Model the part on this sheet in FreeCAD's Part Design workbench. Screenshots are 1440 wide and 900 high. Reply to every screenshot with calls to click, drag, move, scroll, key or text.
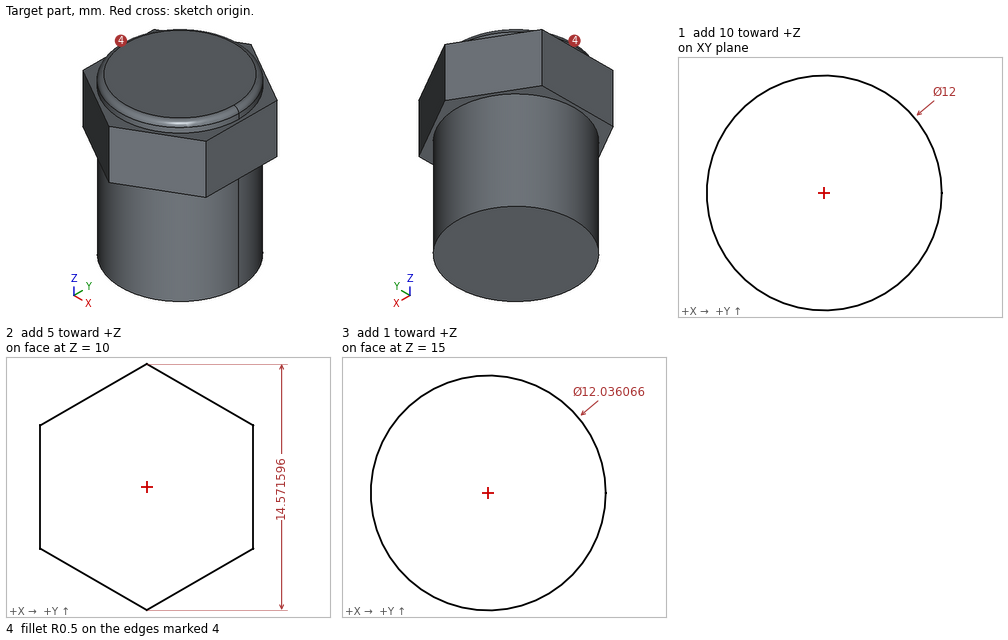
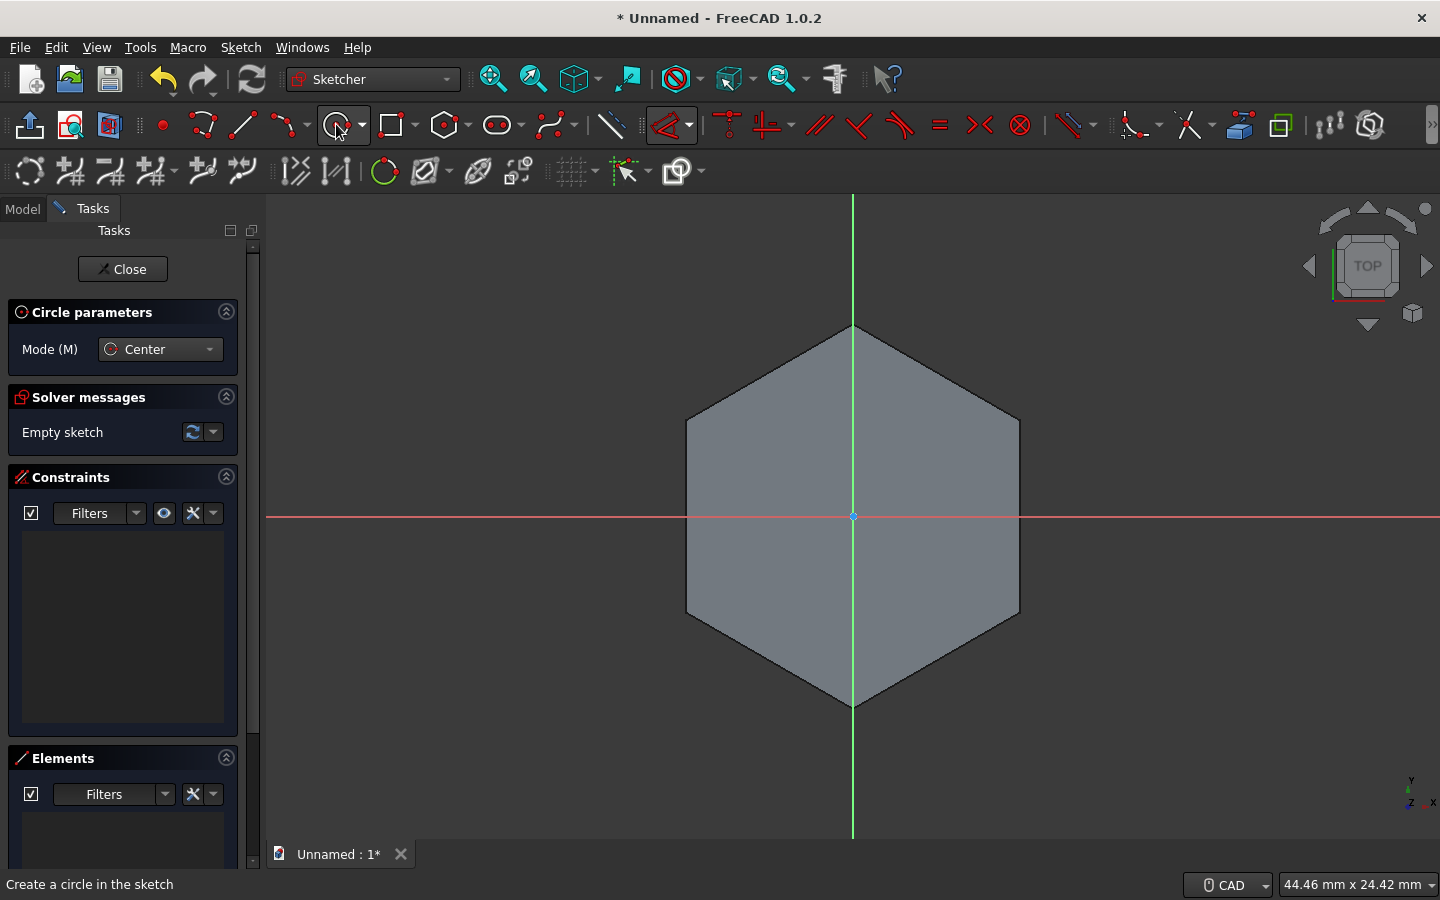
click(853, 516)
click(965, 404)
key(Escape)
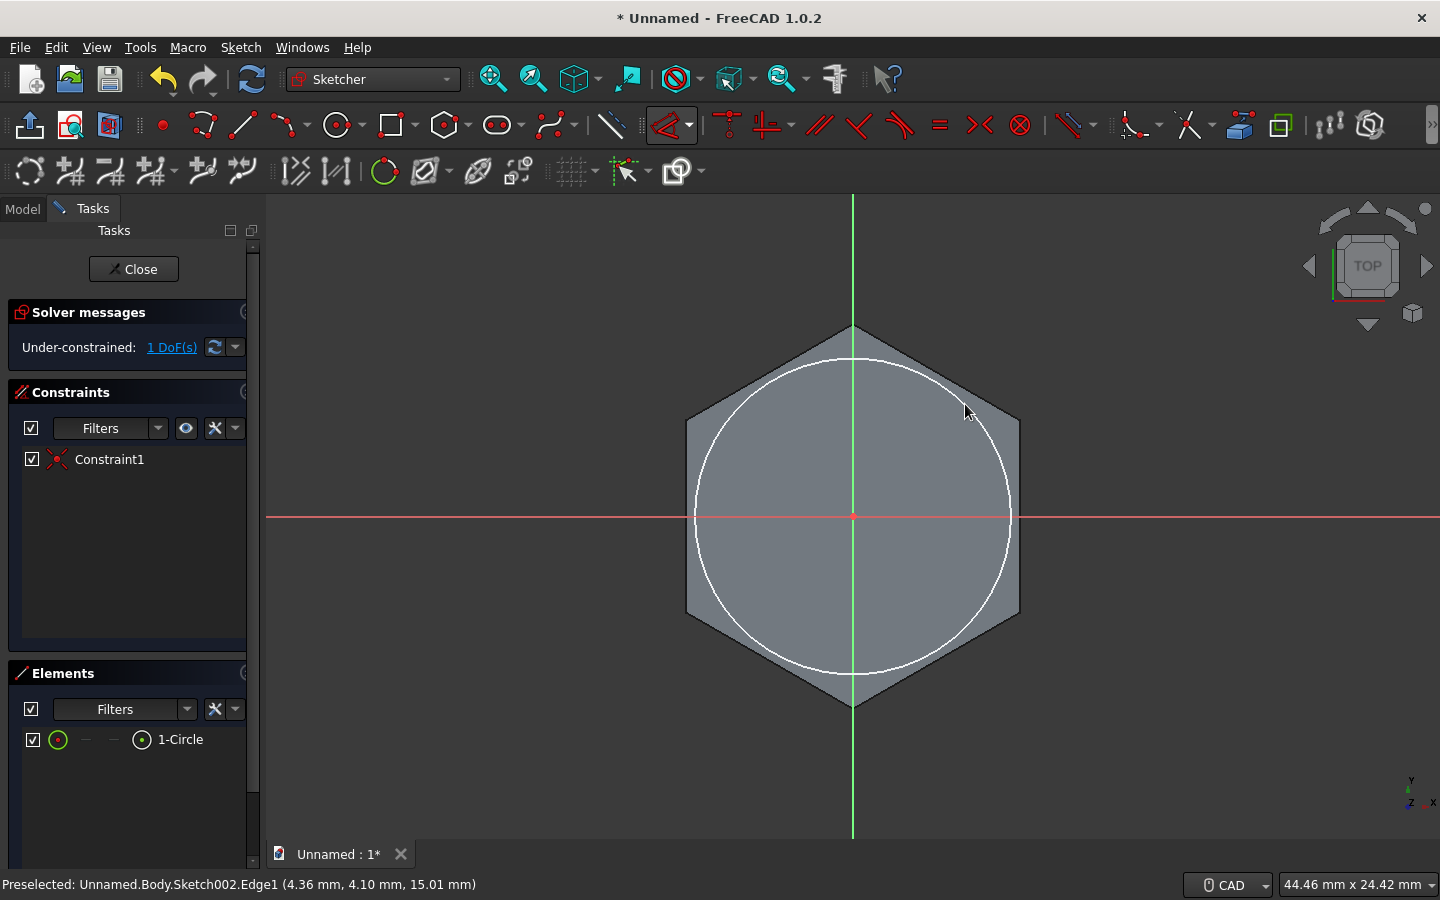
click(964, 404)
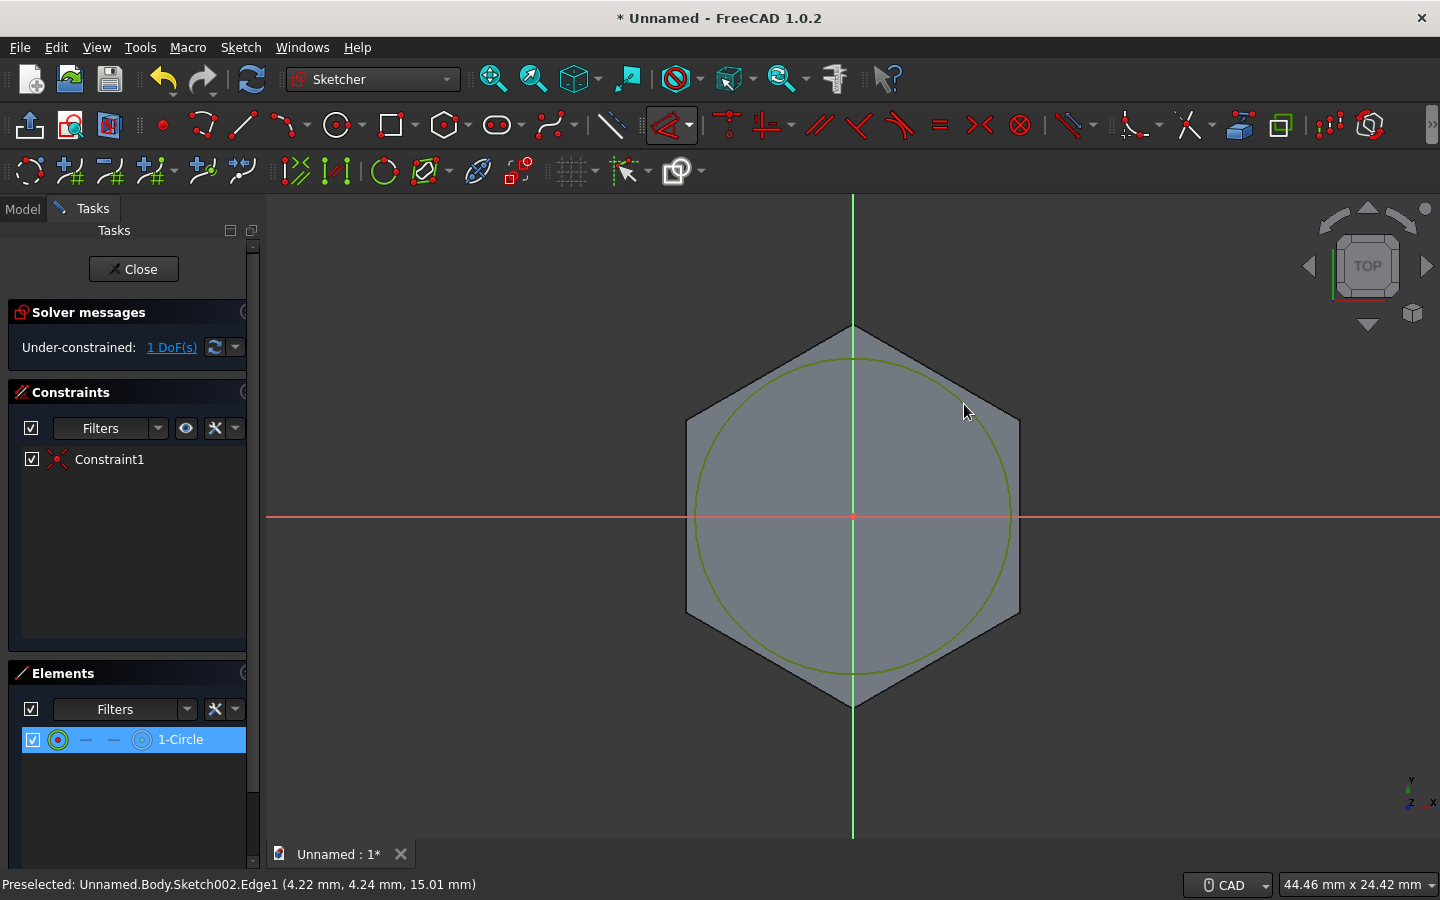
click(692, 126)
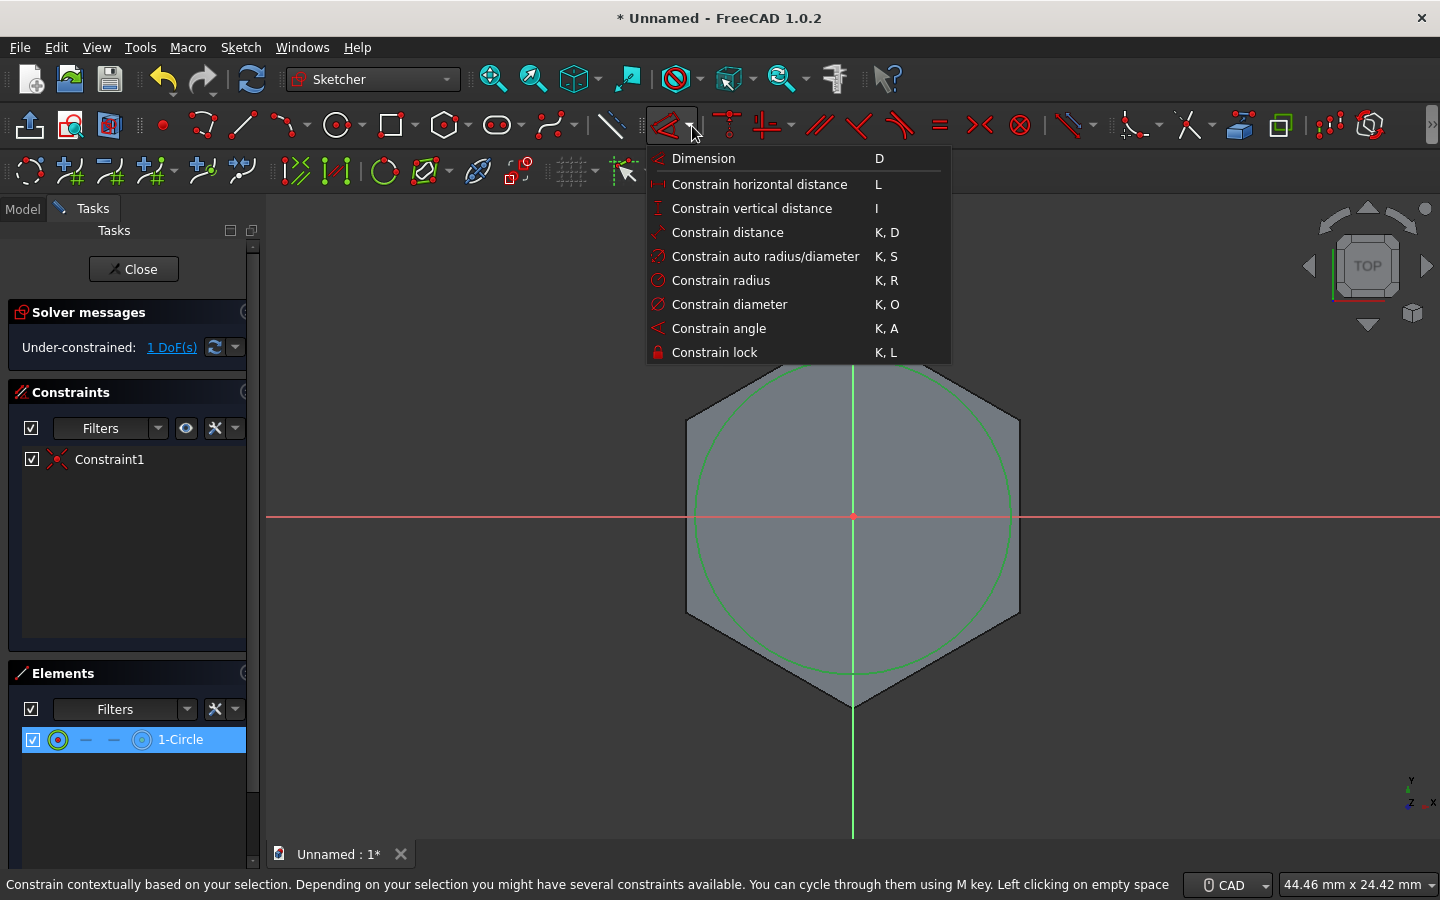
click(799, 304)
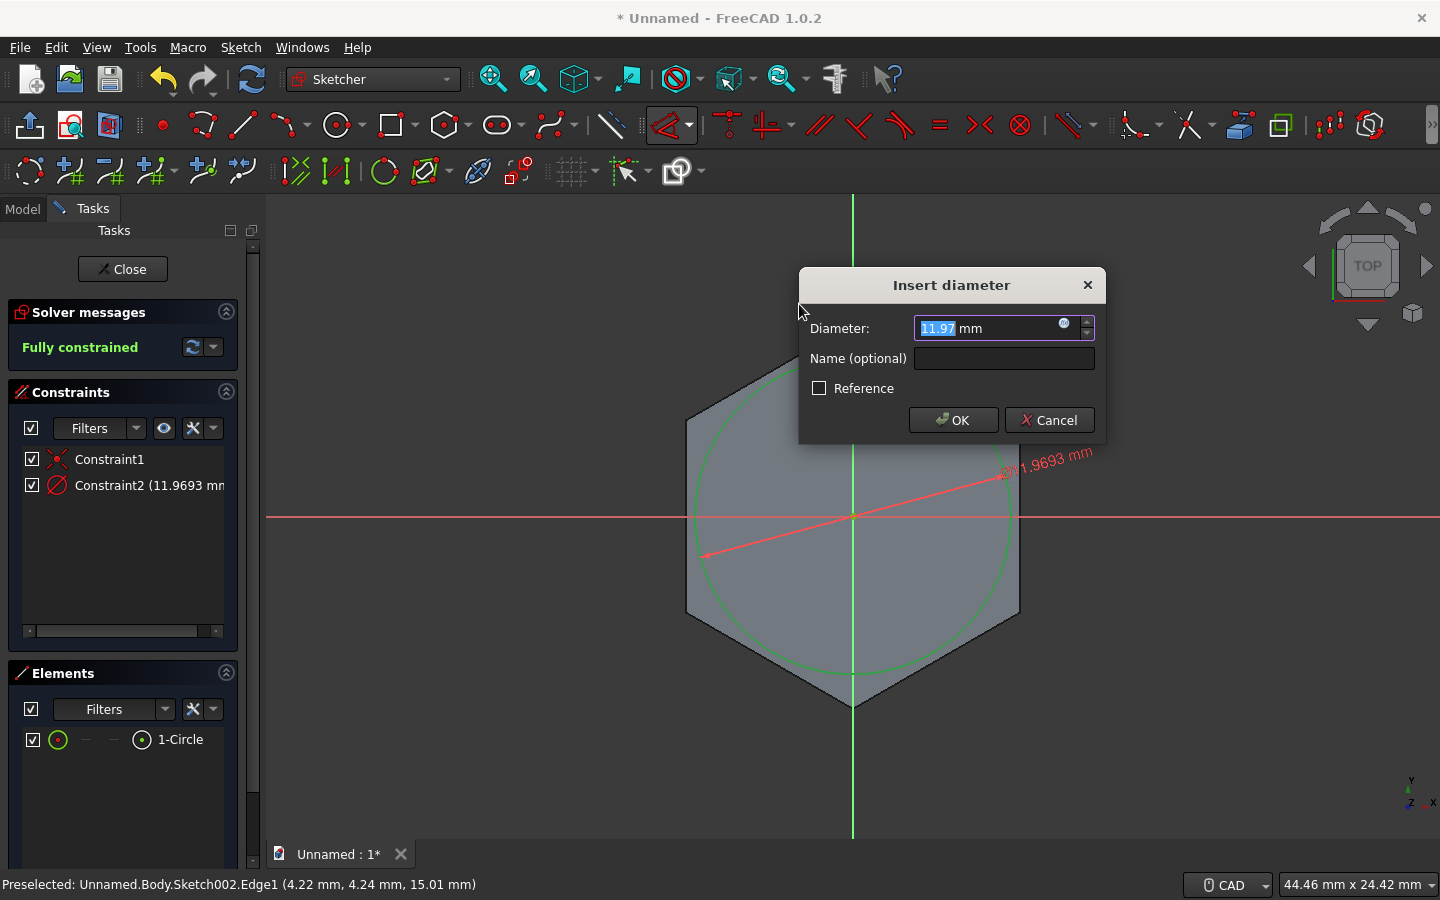
text(12.036066)
key(Return)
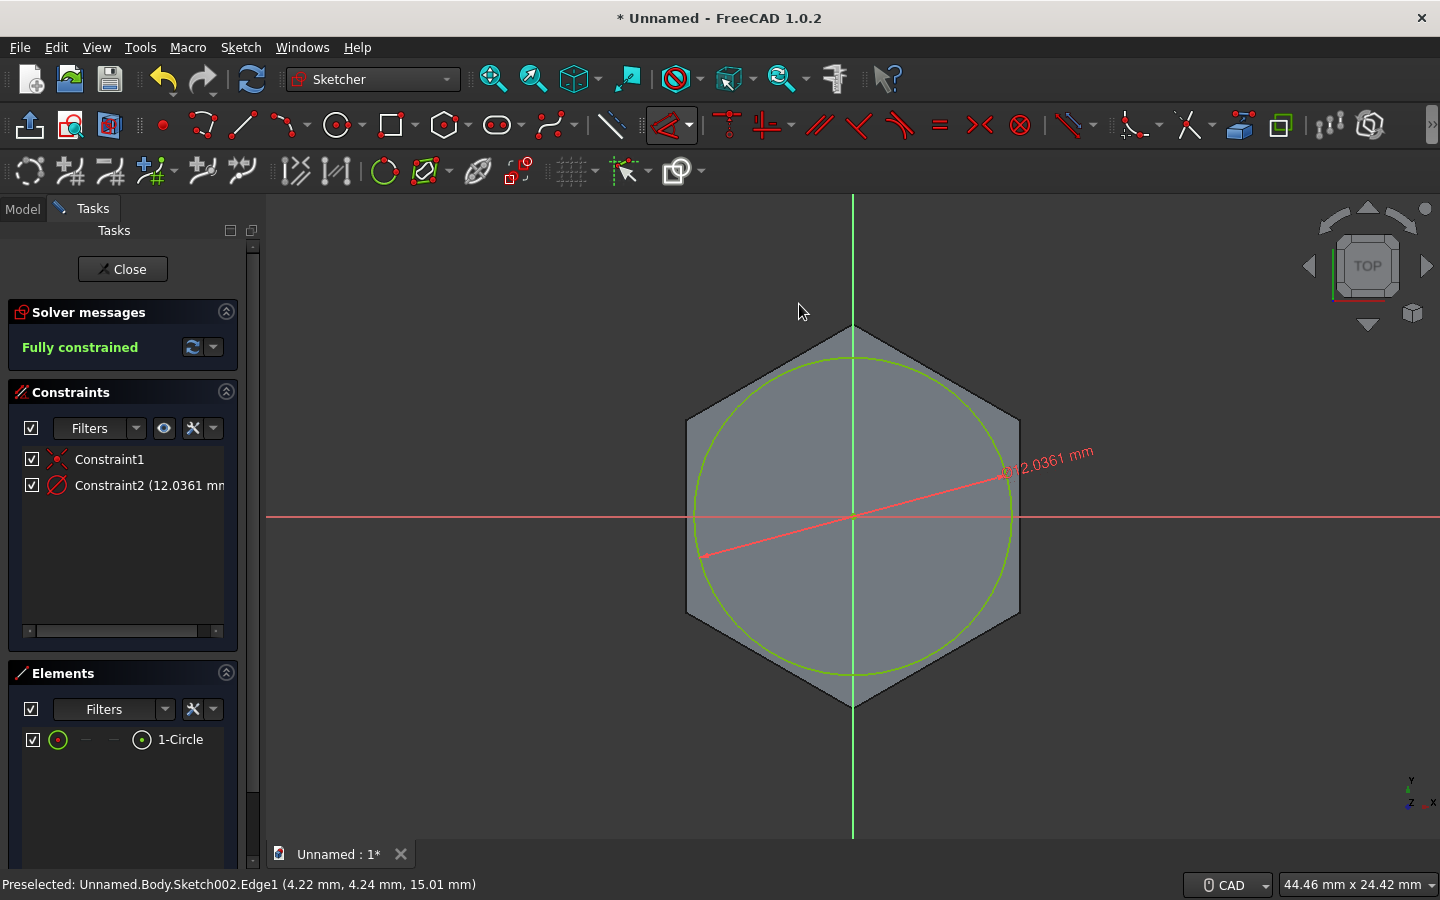
click(123, 269)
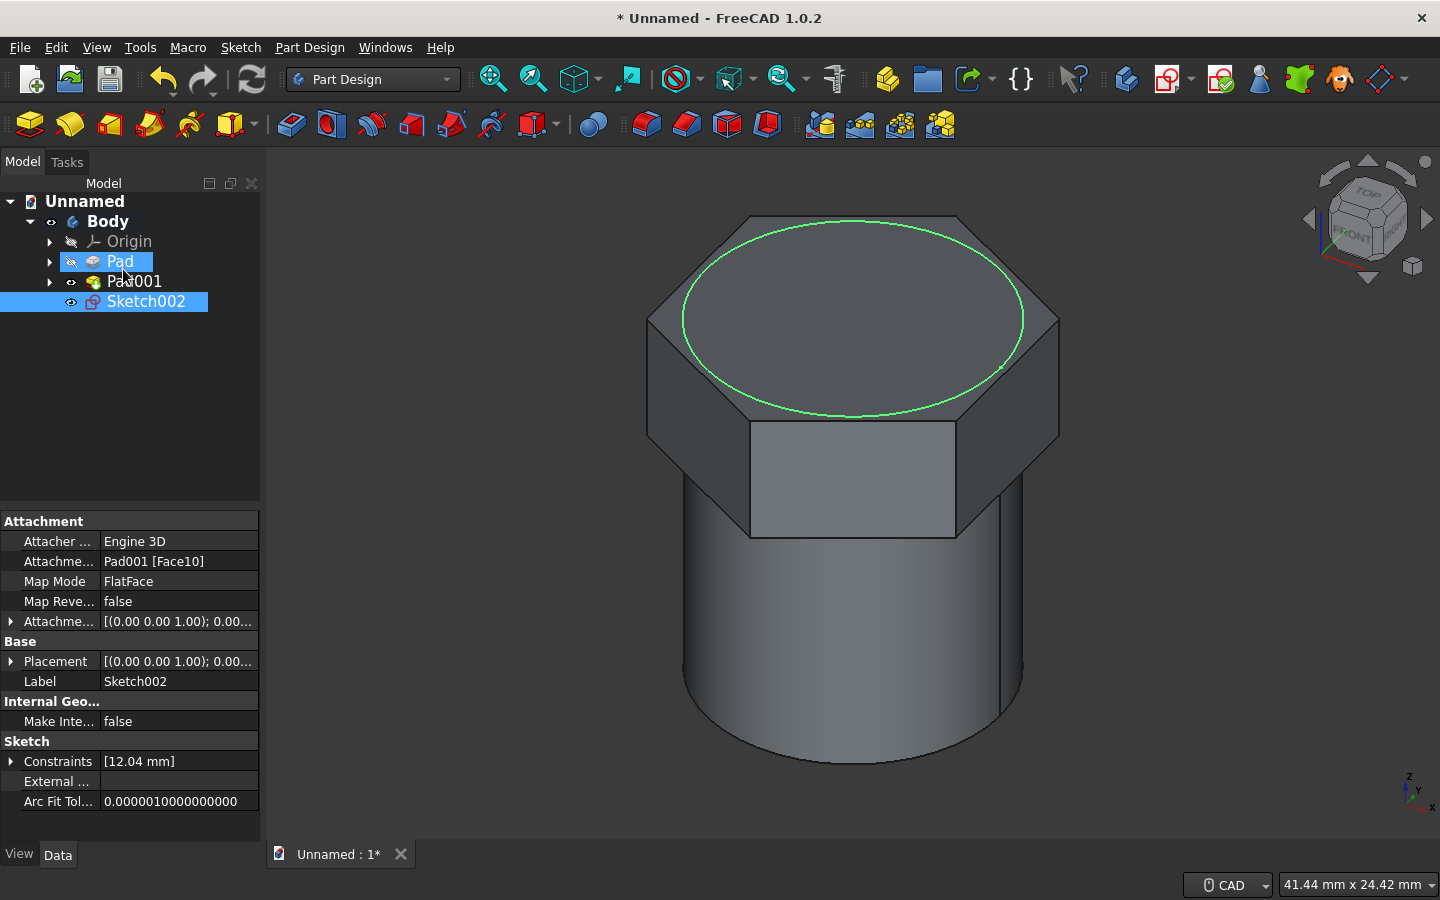
click(30, 124)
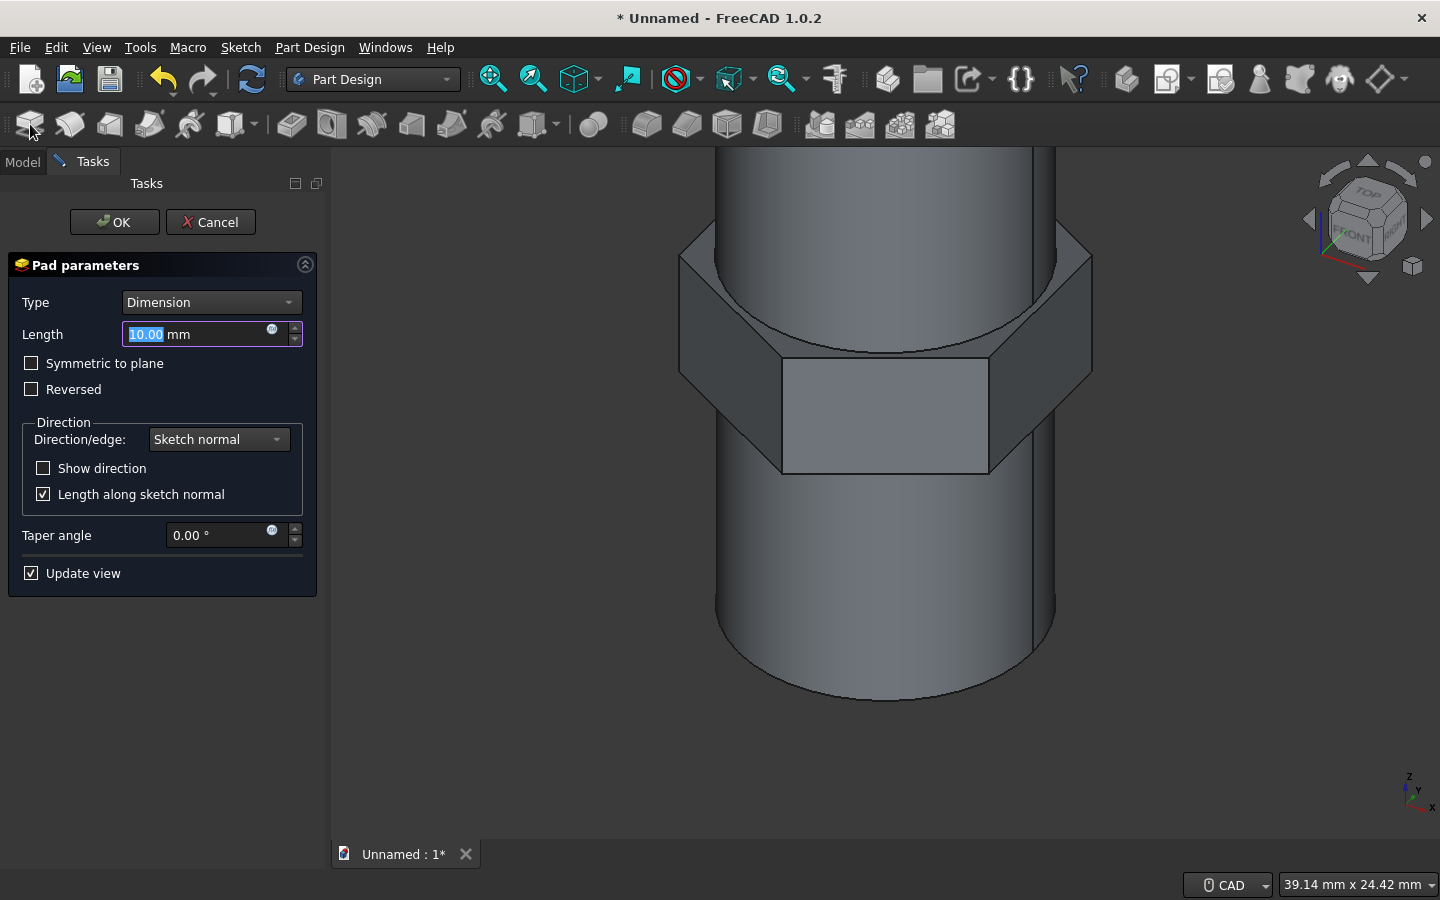
text(1)
key(Tab)